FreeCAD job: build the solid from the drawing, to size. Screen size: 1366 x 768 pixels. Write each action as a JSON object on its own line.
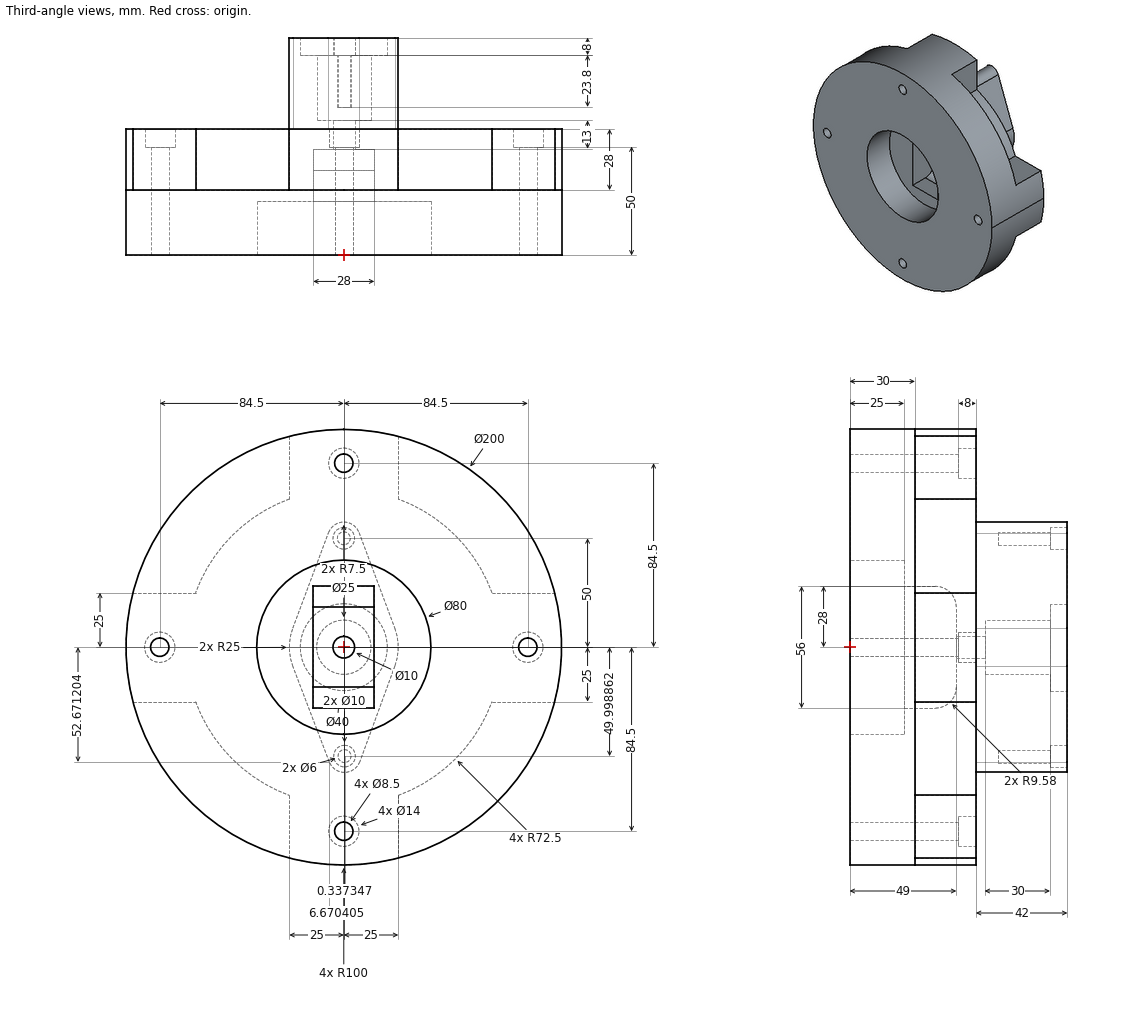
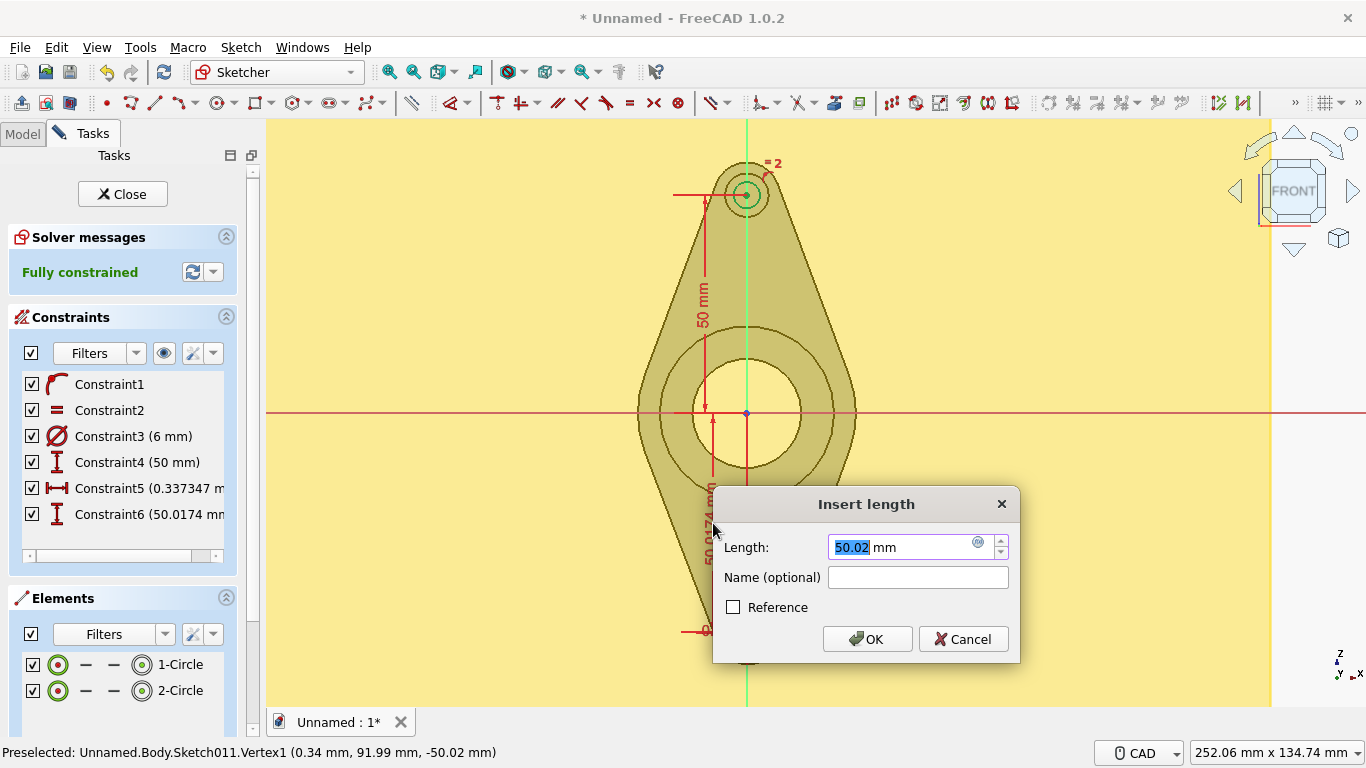
{"action": "type", "text": "49.998862"}
{"action": "key", "text": "Return"}
{"action": "key", "text": "Escape"}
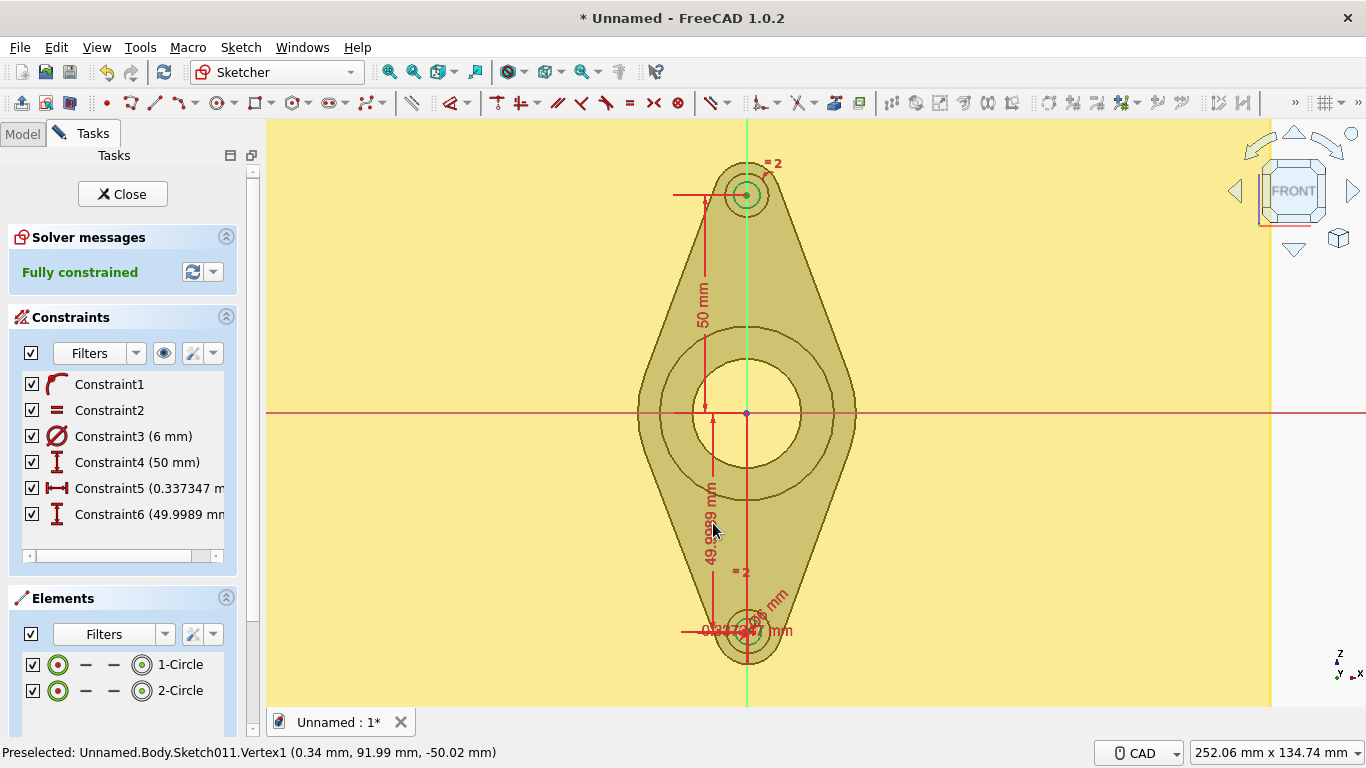
{"action": "left_click", "coordinate": [123, 194]}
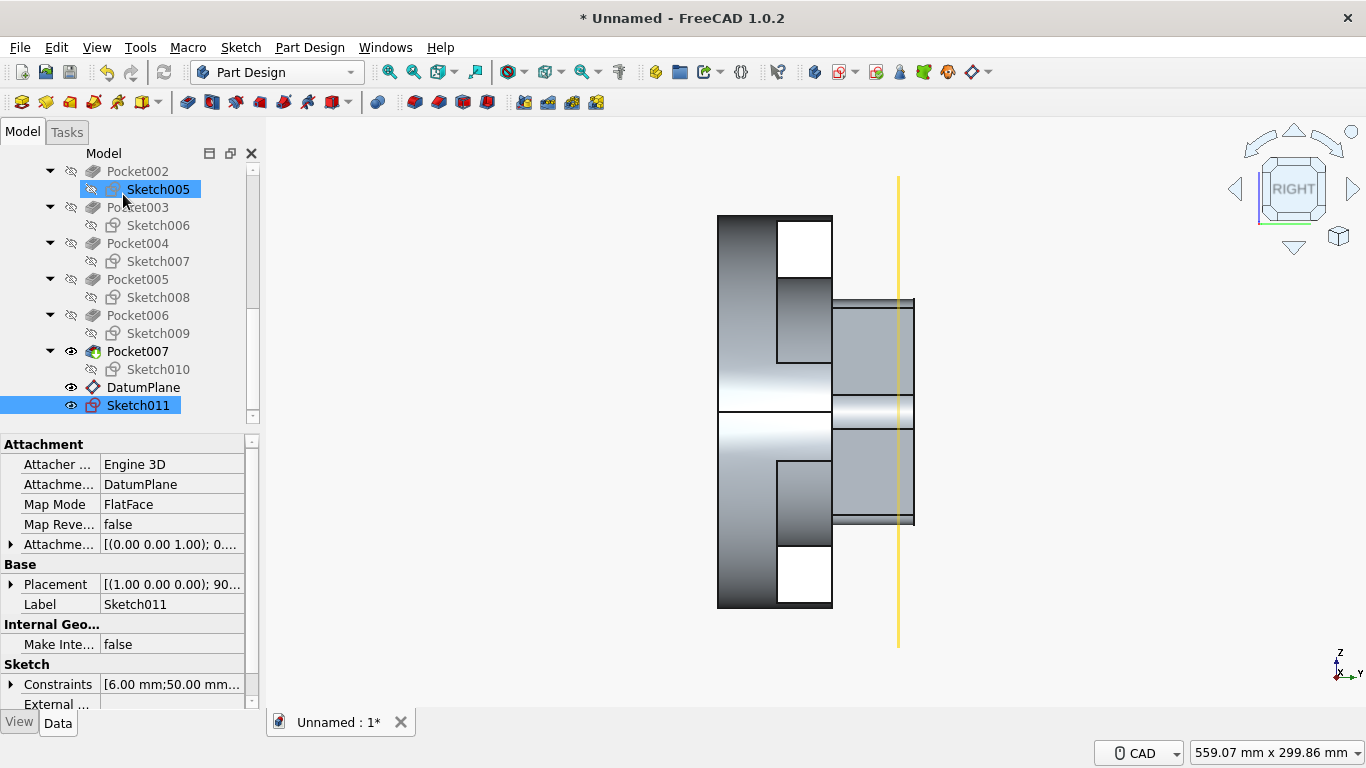
{"action": "left_click", "coordinate": [188, 102]}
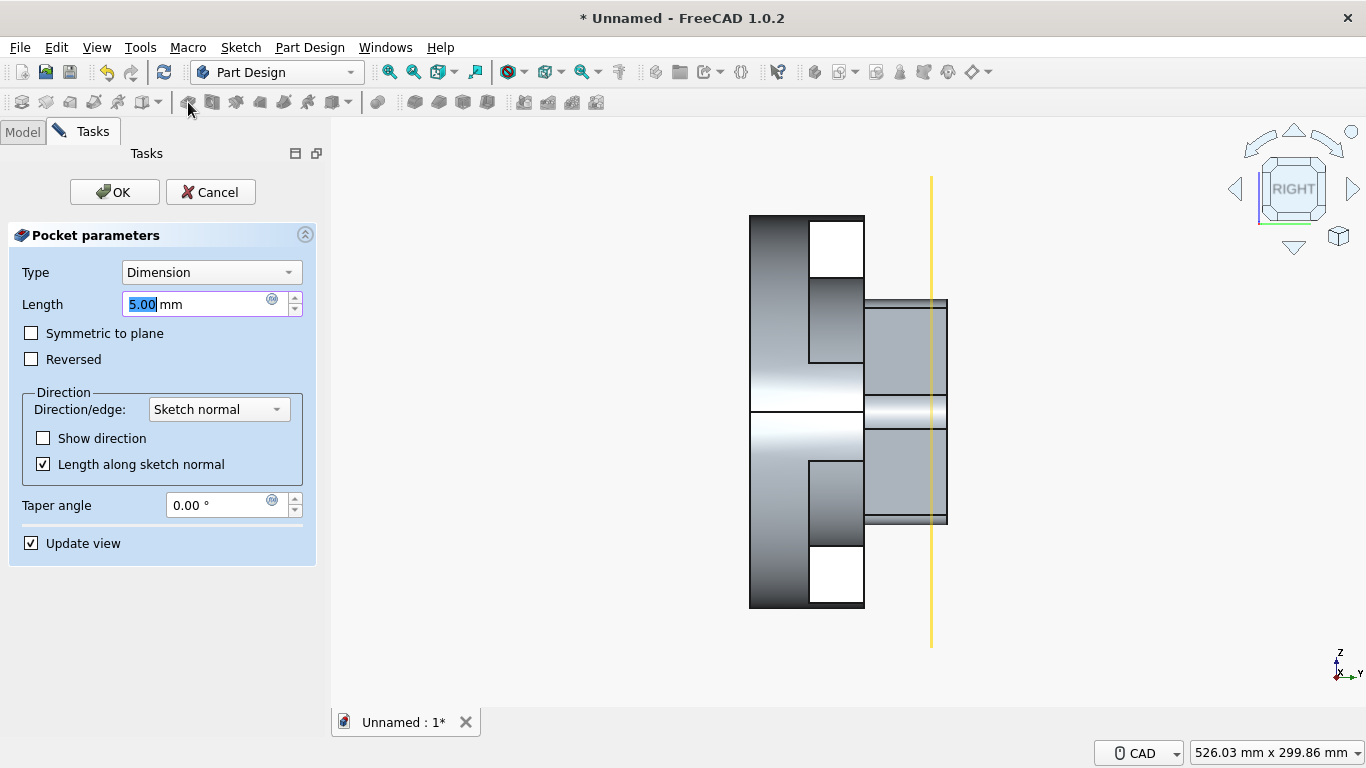
{"action": "type", "text": "23.8"}
{"action": "key", "text": "Tab"}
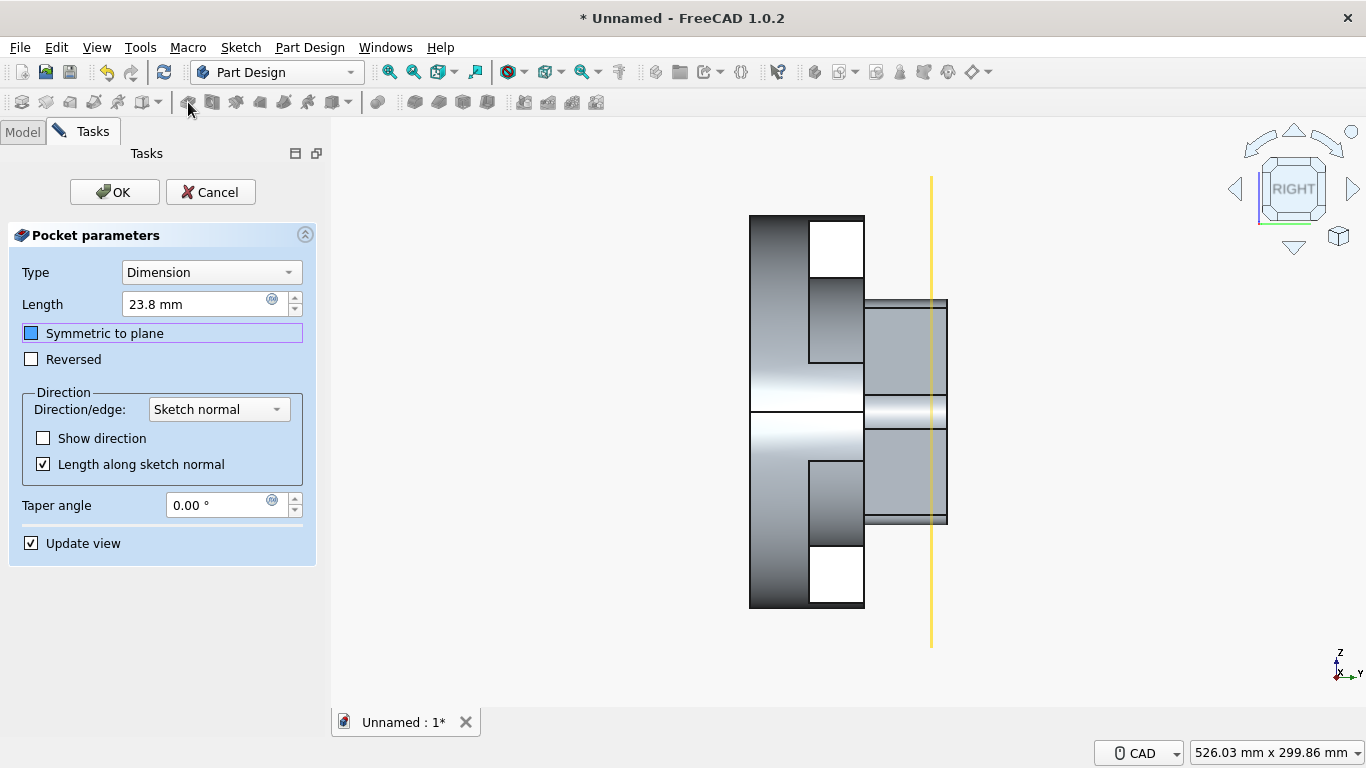
{"action": "left_click", "coordinate": [30, 359]}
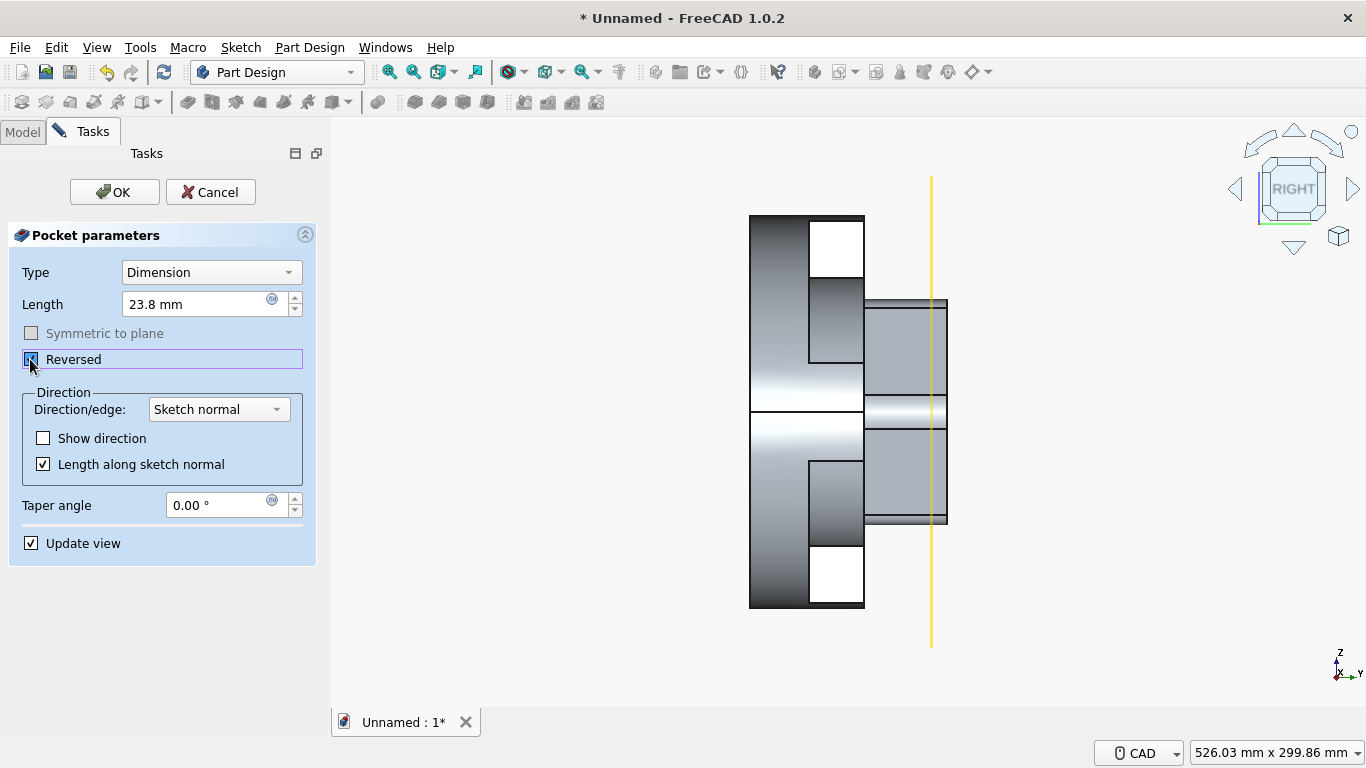
{"action": "left_click", "coordinate": [115, 192]}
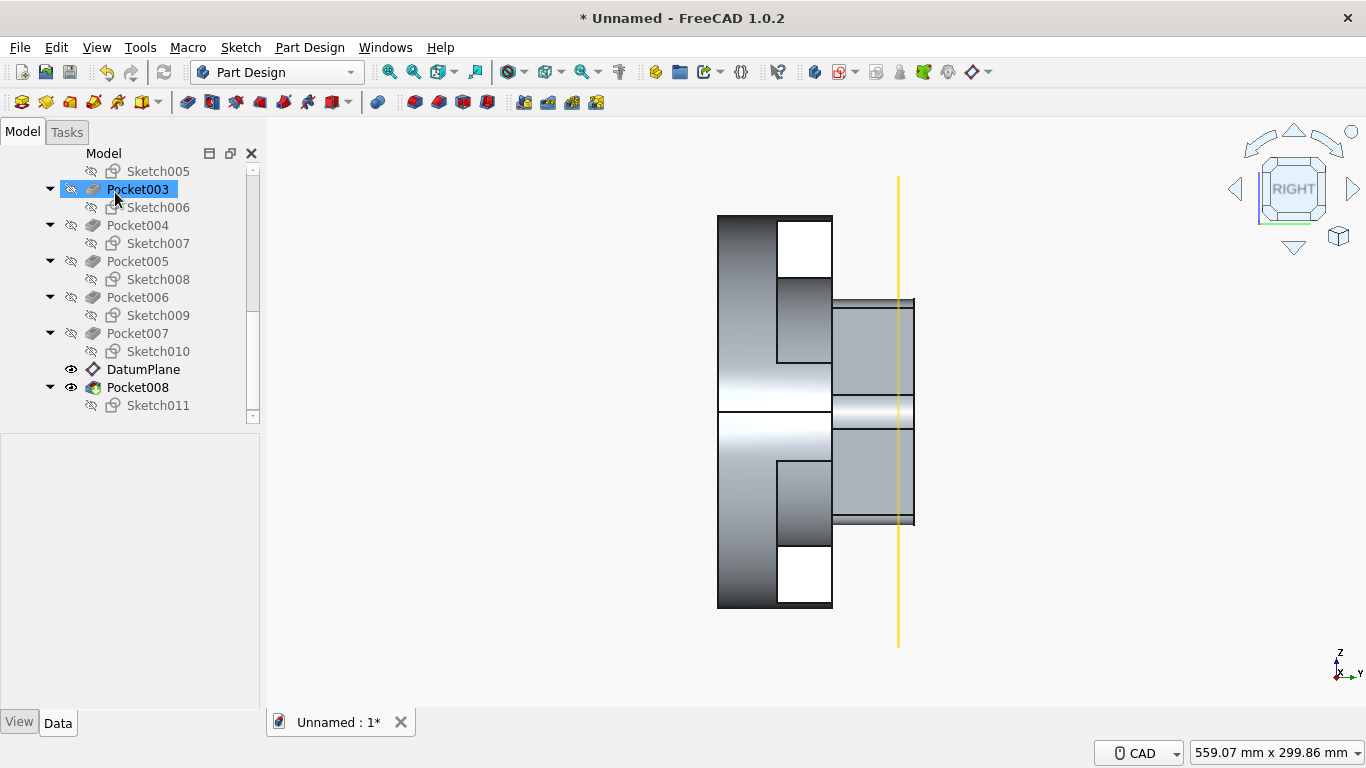
{"action": "left_click", "coordinate": [116, 369]}
{"action": "key", "text": "space"}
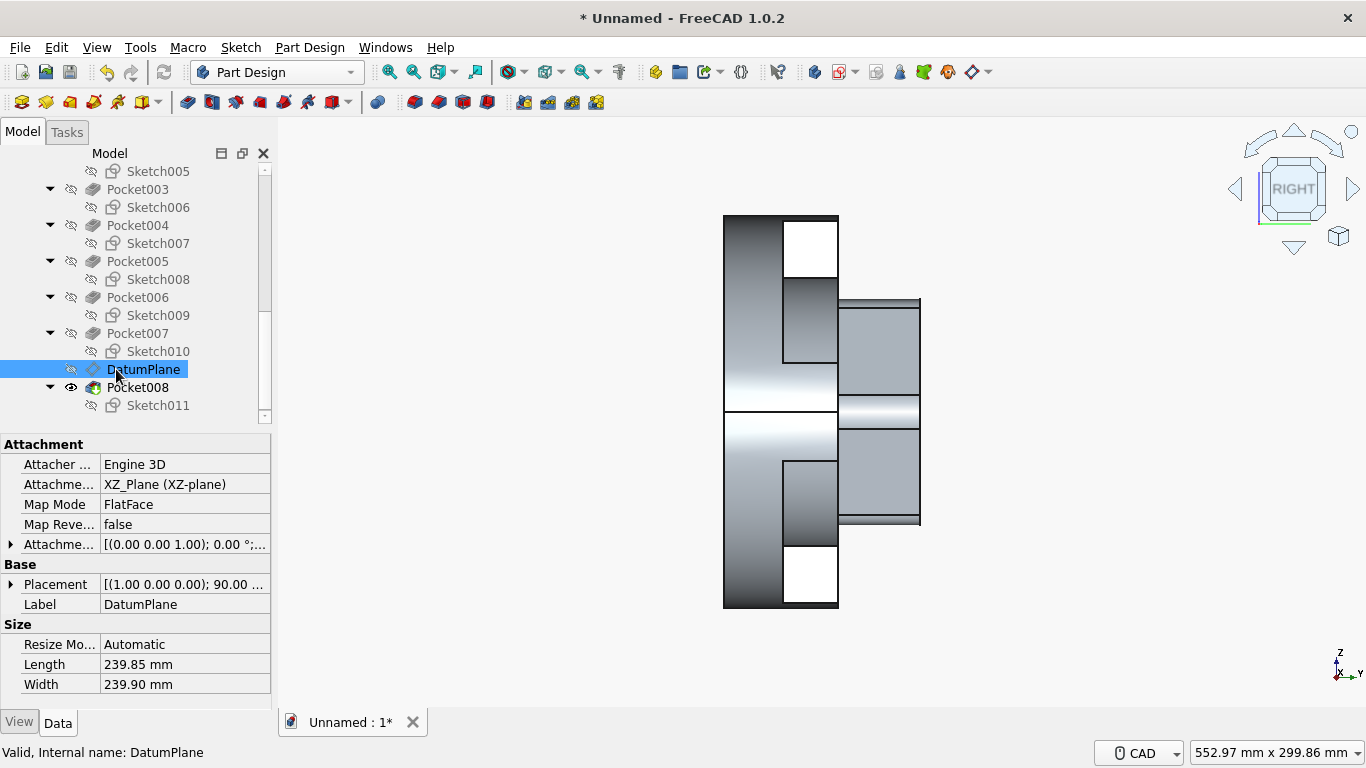
{"action": "key", "text": "0"}